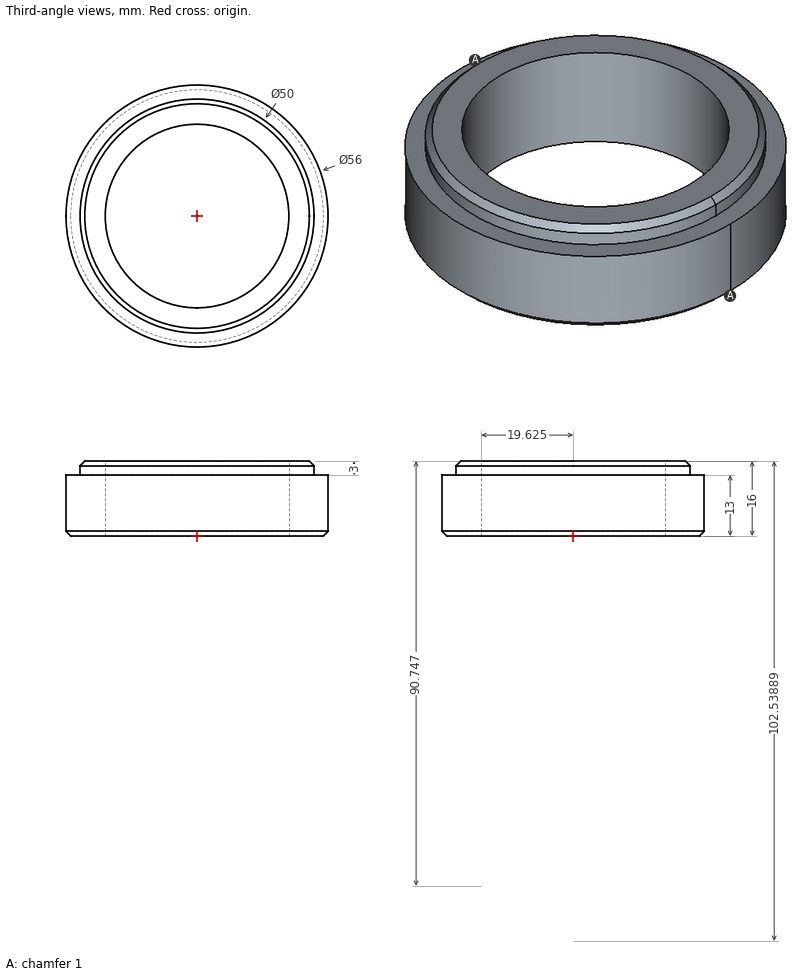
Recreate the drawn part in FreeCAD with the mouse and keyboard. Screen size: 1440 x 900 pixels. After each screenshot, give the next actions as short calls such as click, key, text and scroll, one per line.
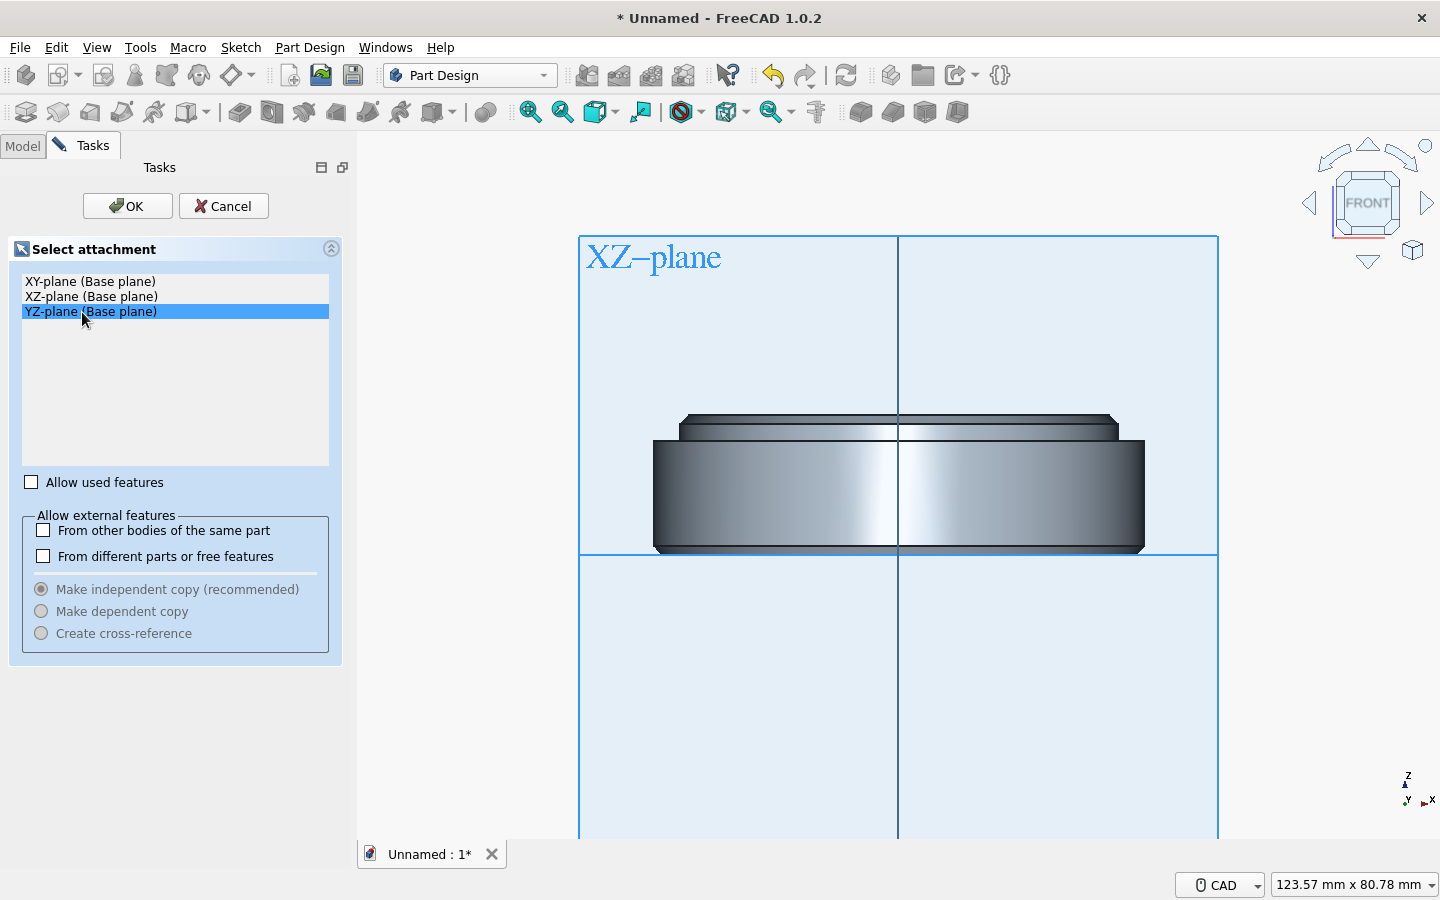
click(128, 206)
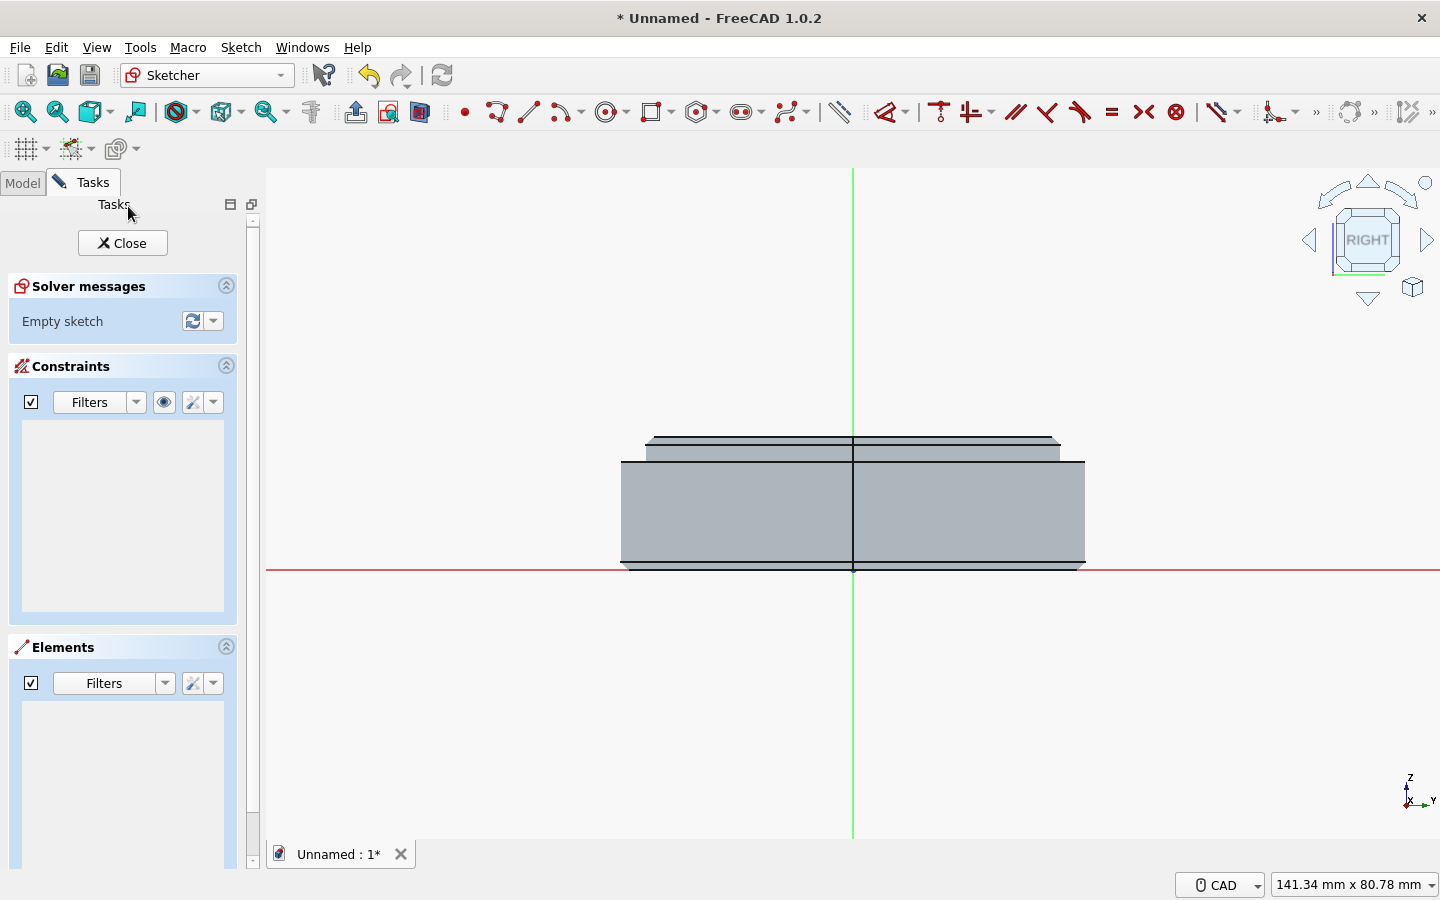
click(420, 112)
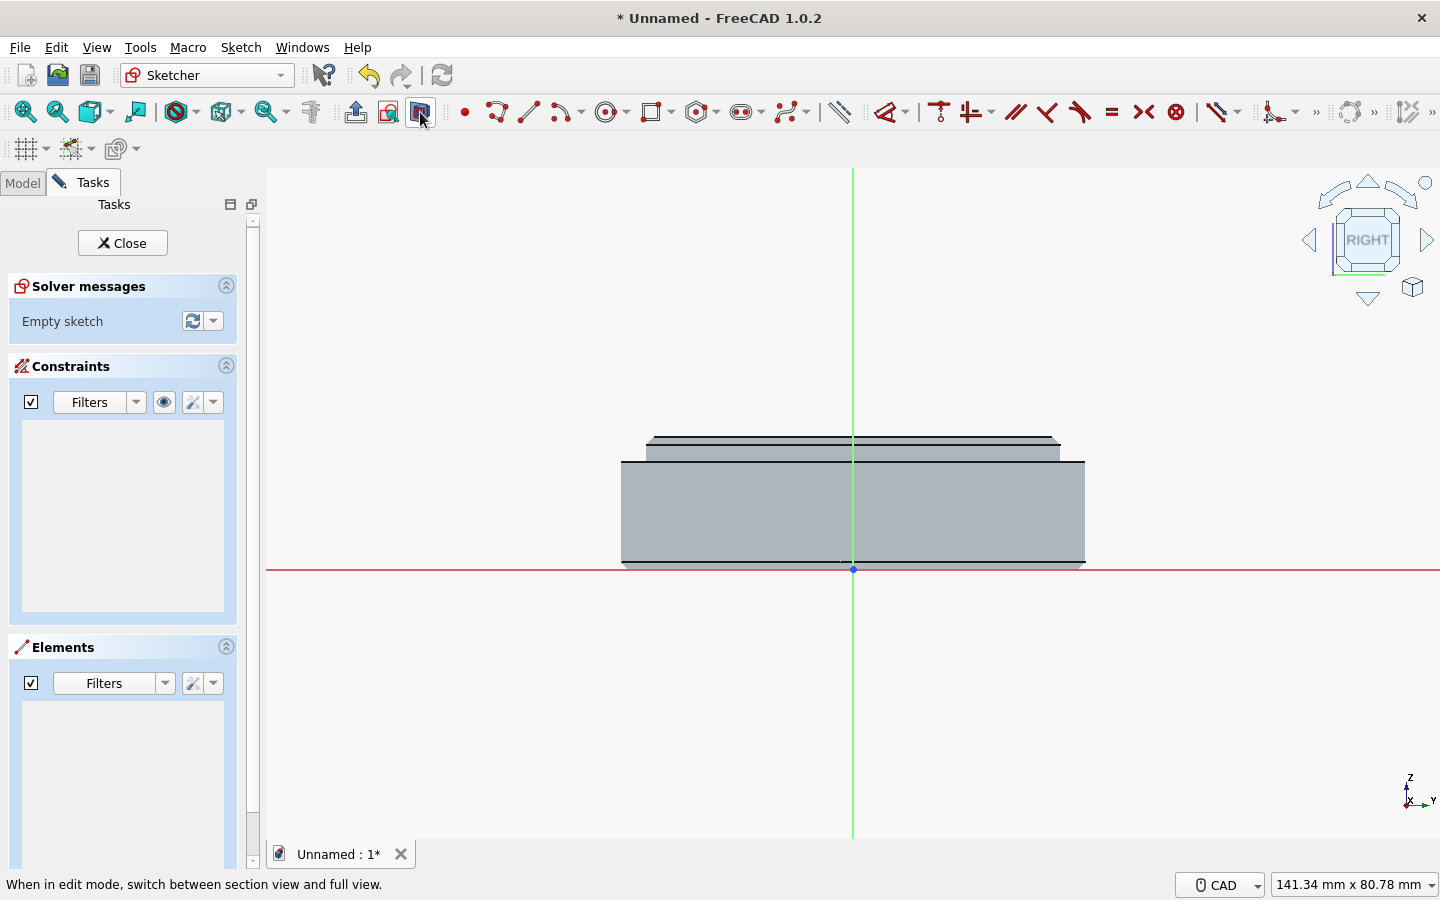
scroll(795, 210, down, 4)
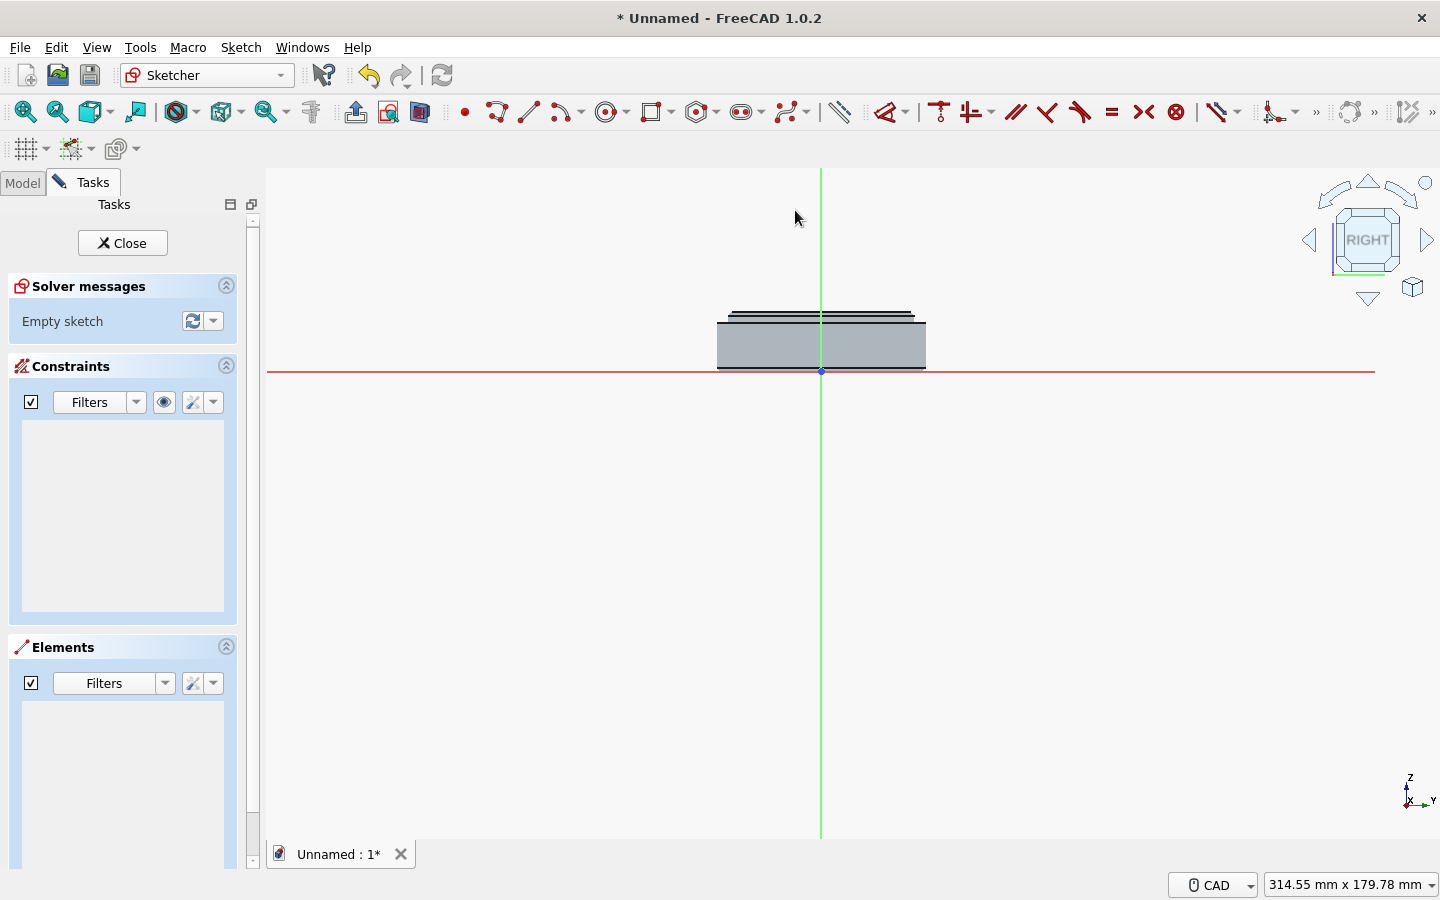
key(g)
key(m)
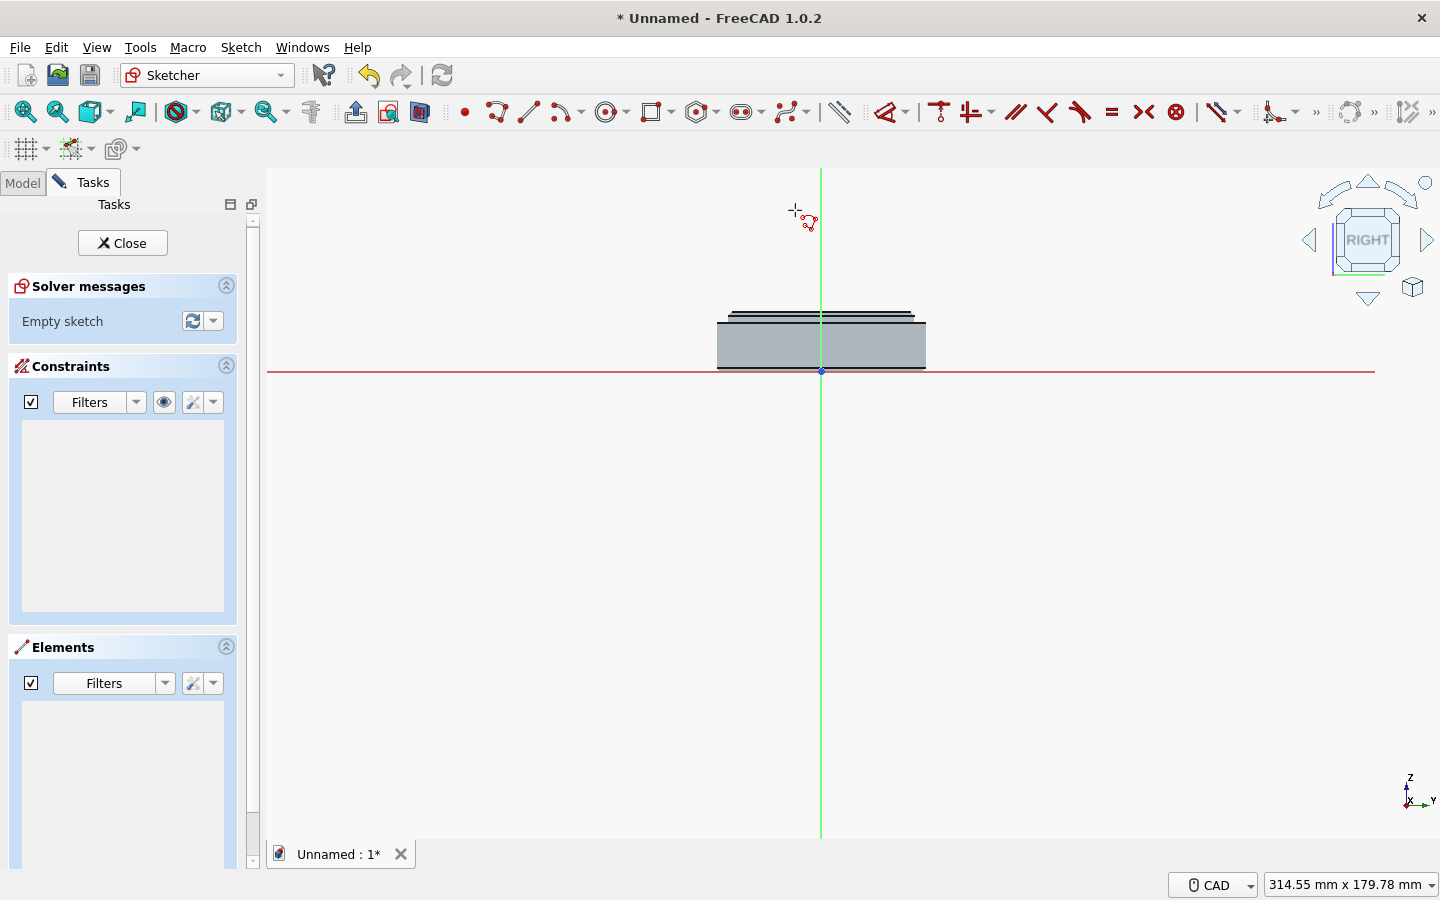
click(821, 312)
click(748, 312)
click(748, 651)
click(812, 695)
click(821, 313)
key(Escape)
key(Escape)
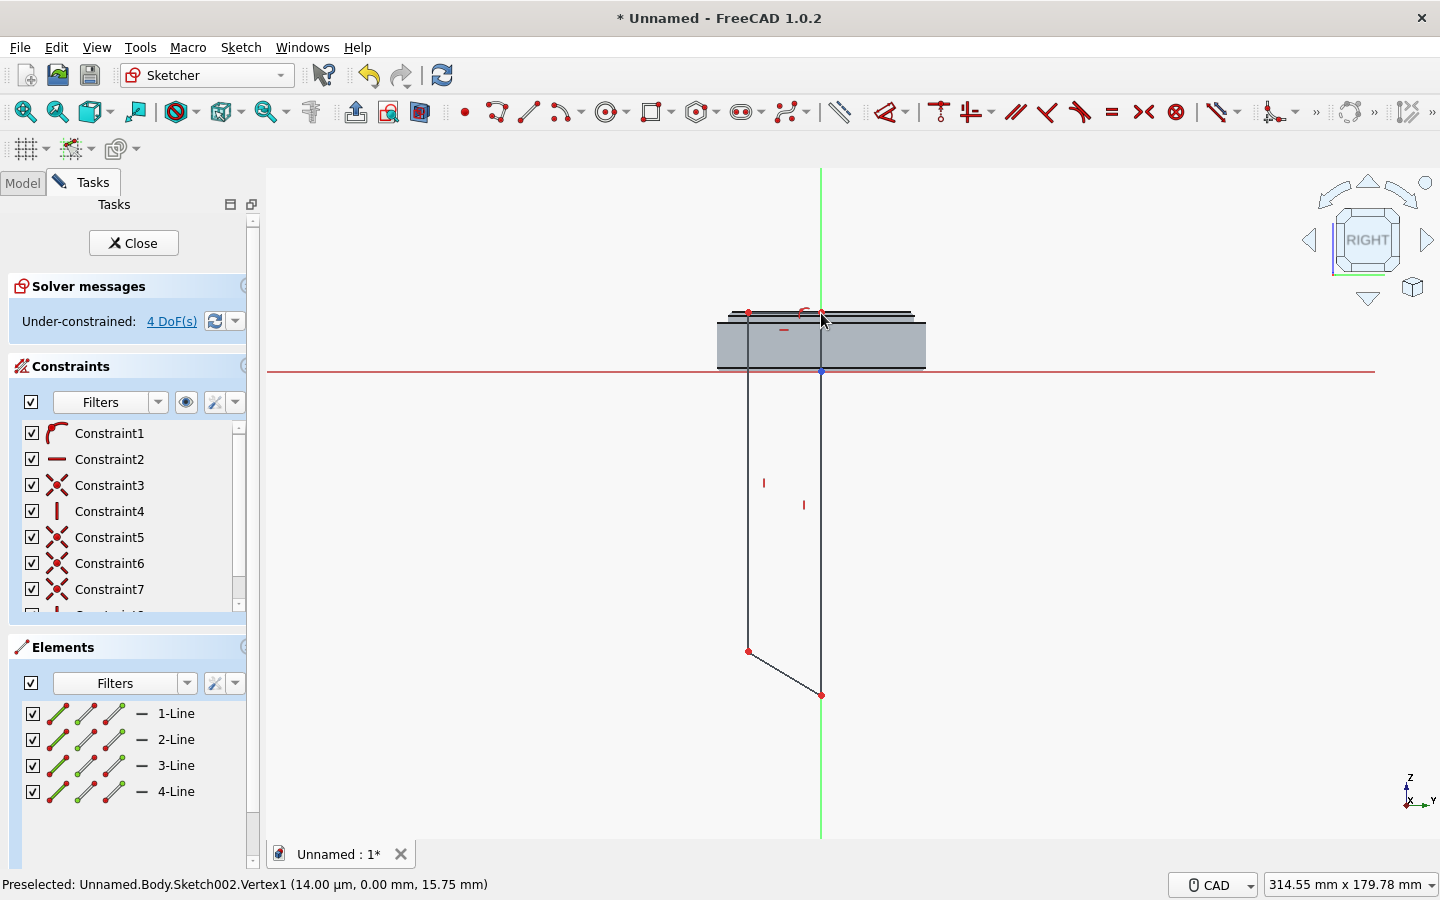
click(821, 313)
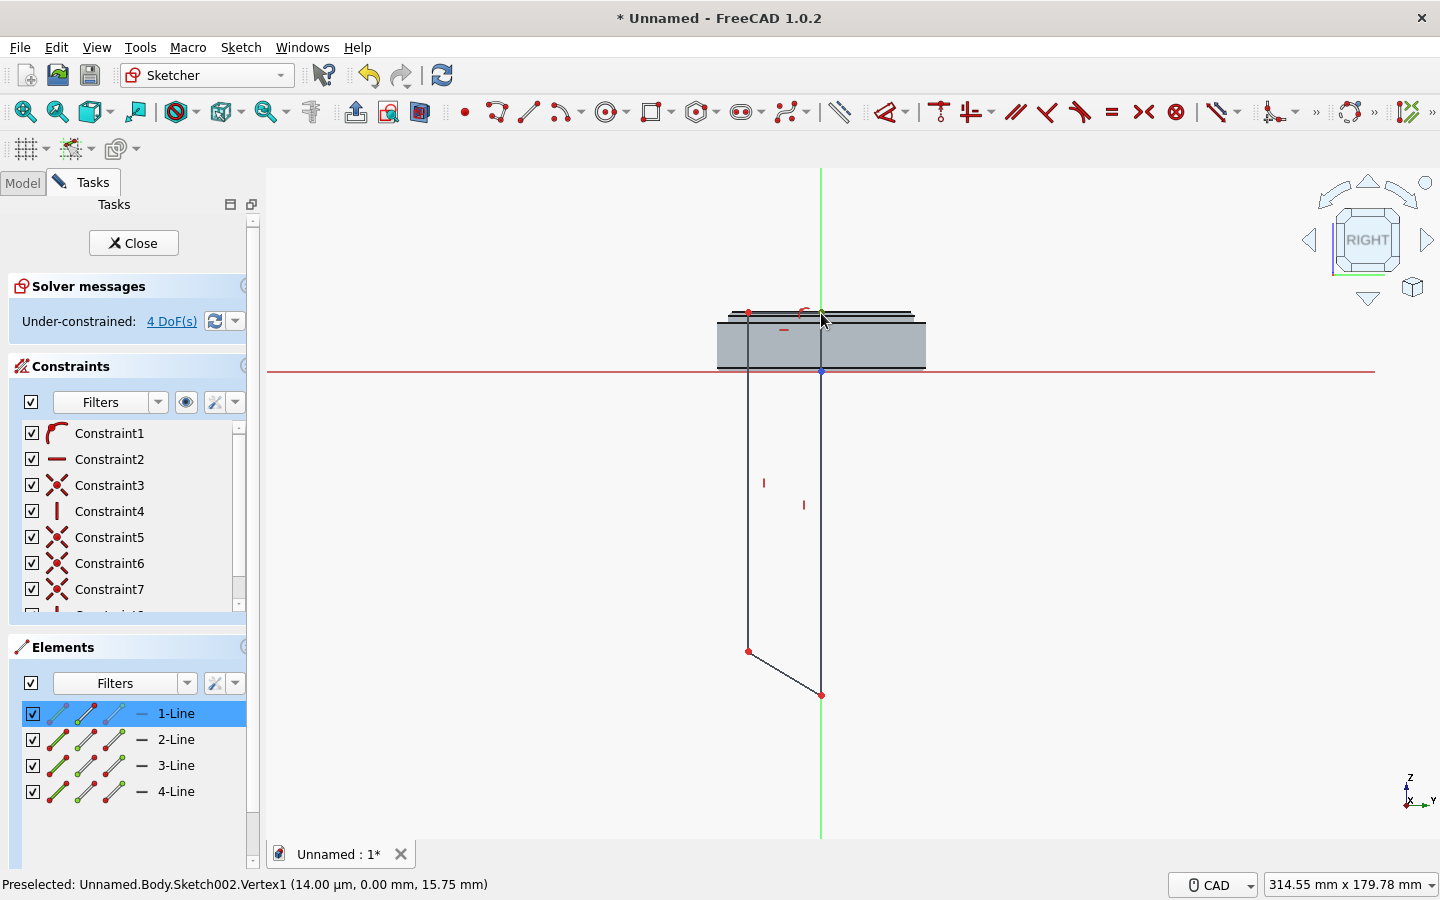
click(908, 112)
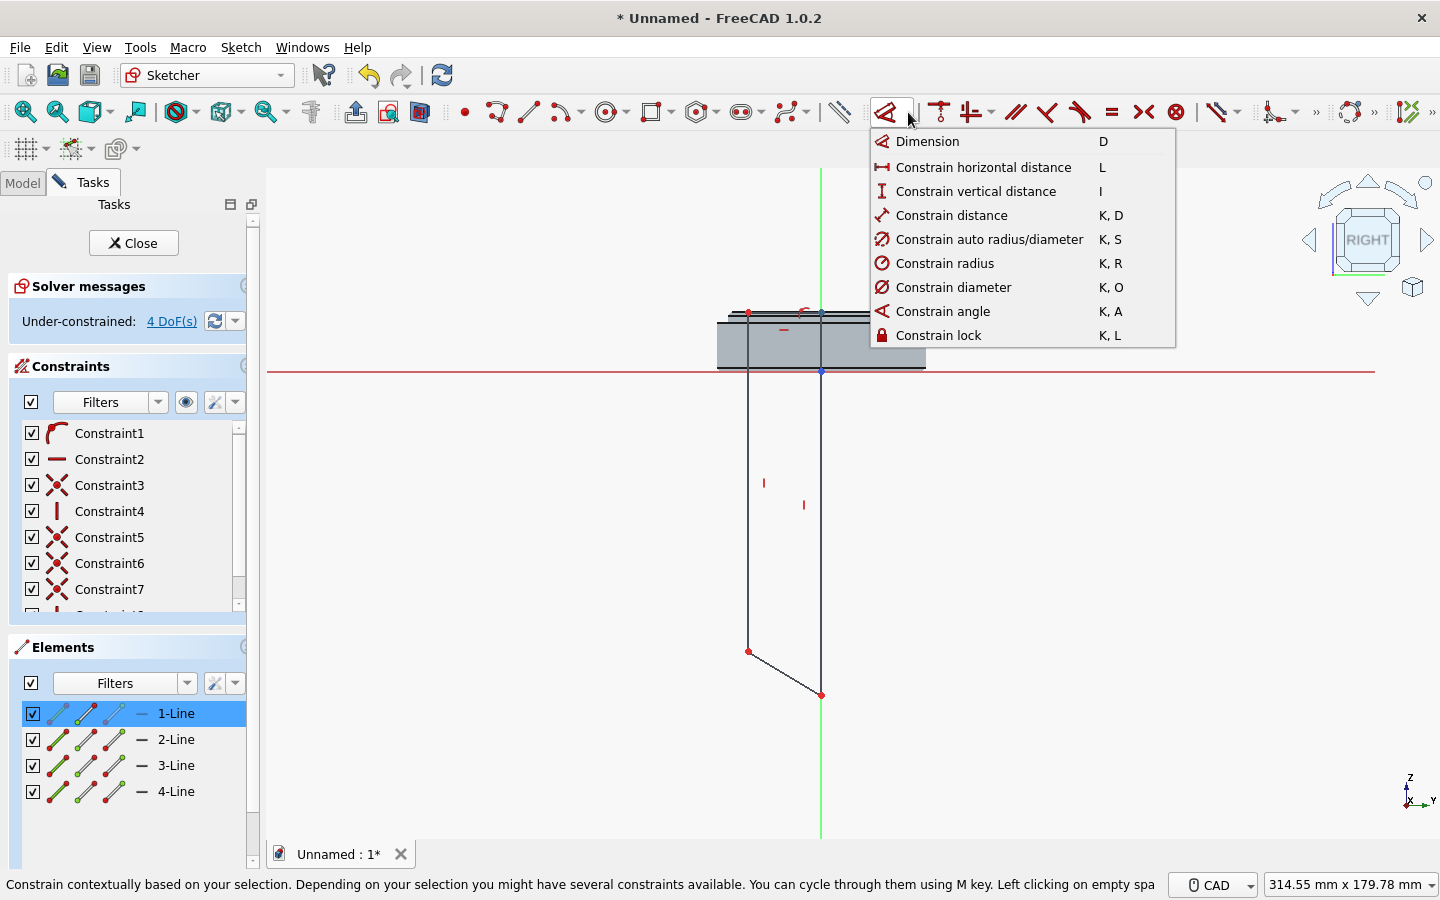
click(1023, 191)